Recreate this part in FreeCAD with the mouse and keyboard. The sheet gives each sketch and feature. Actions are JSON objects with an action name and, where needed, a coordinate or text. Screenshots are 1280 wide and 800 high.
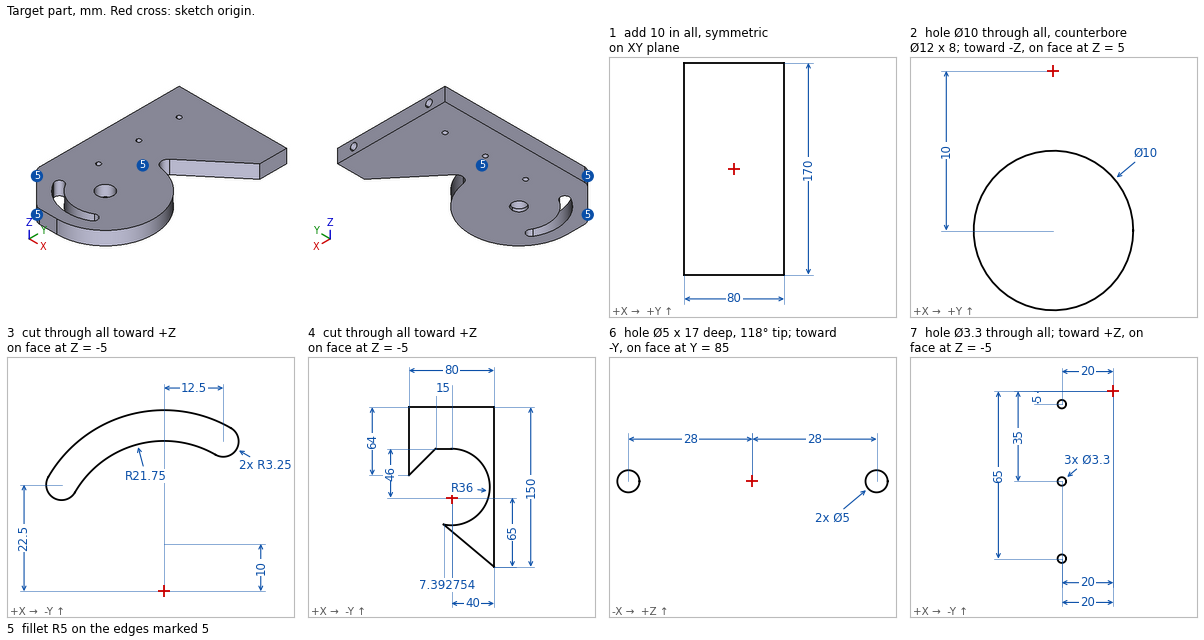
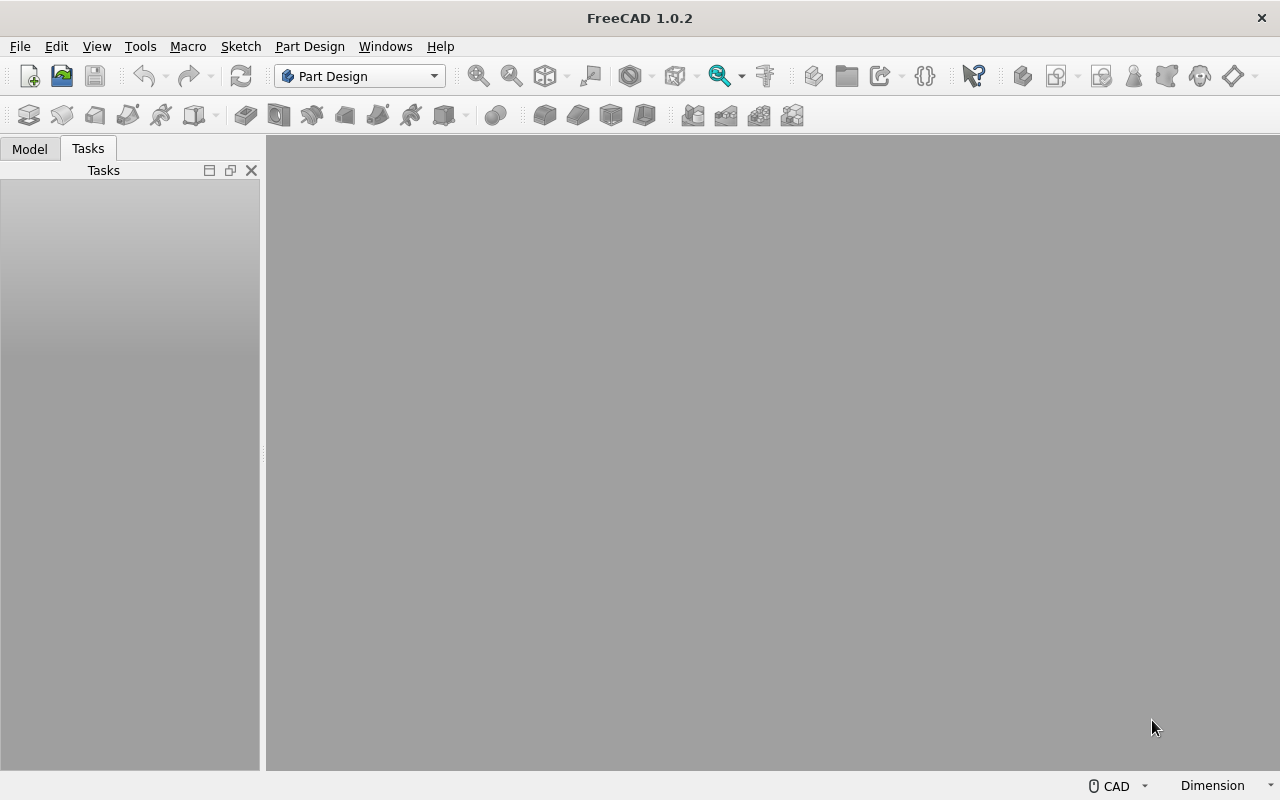
{"action": "key", "text": "ctrl+n"}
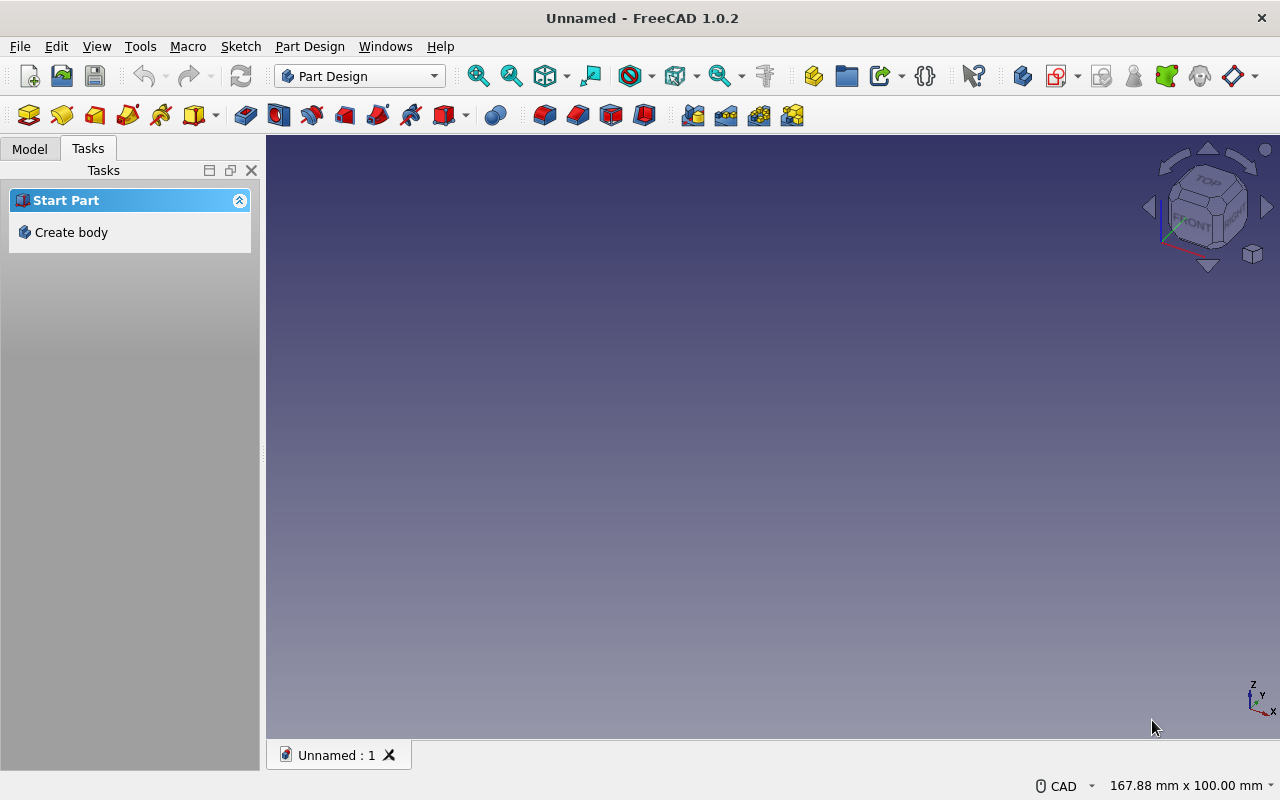
{"action": "left_click", "coordinate": [1056, 76]}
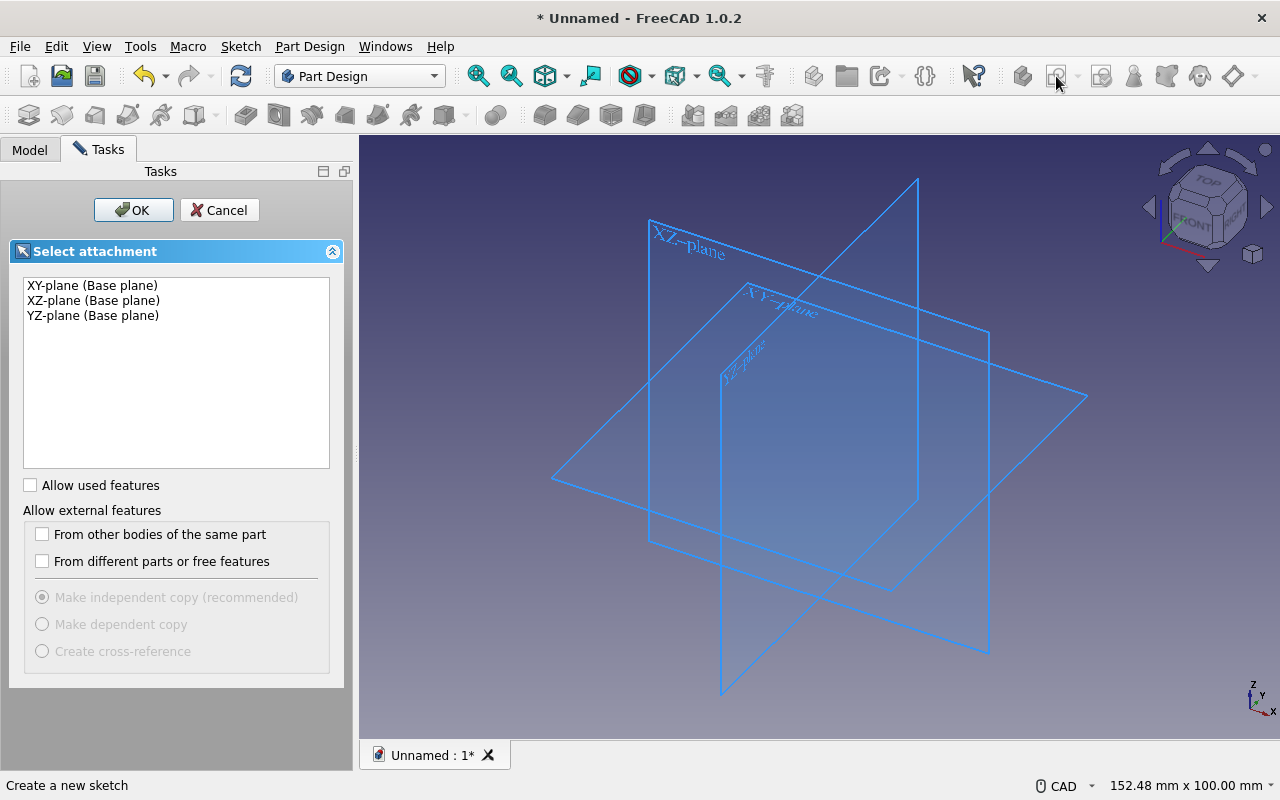
{"action": "left_click", "coordinate": [84, 286]}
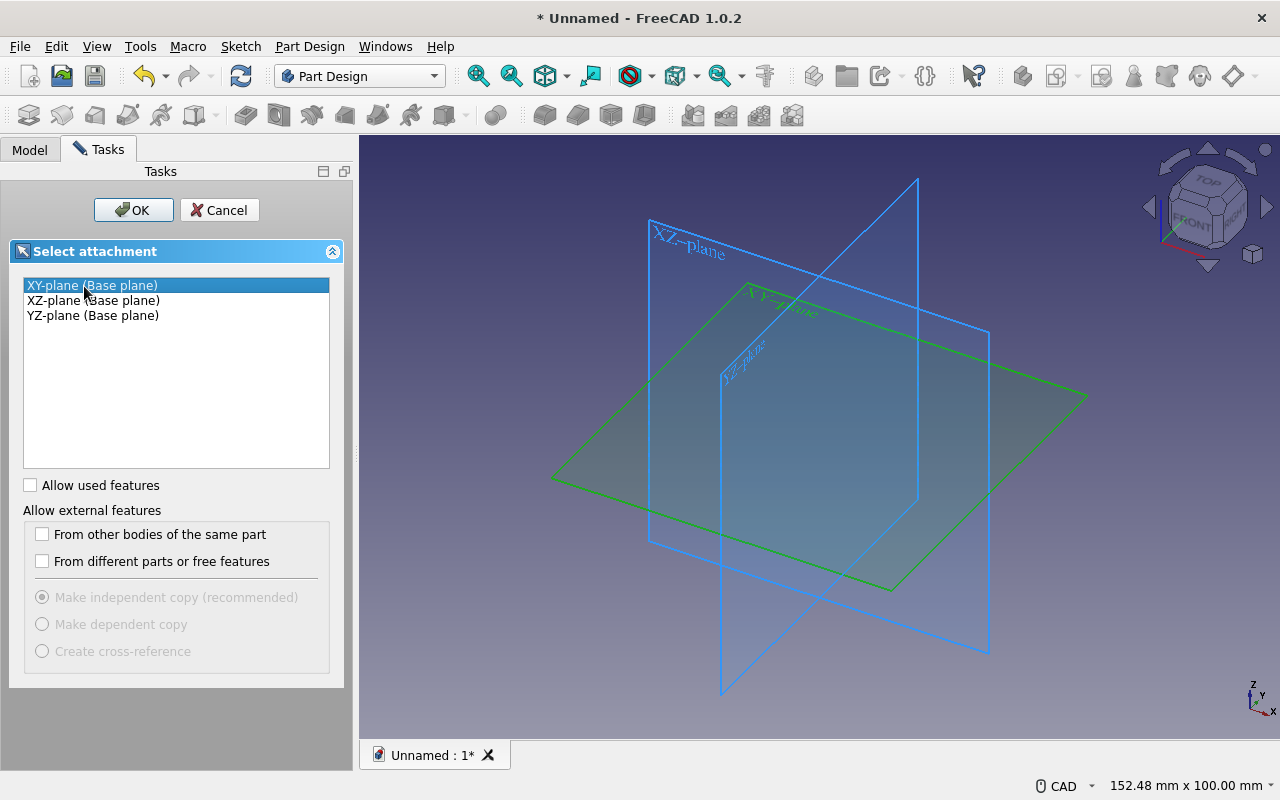
{"action": "left_click", "coordinate": [134, 210]}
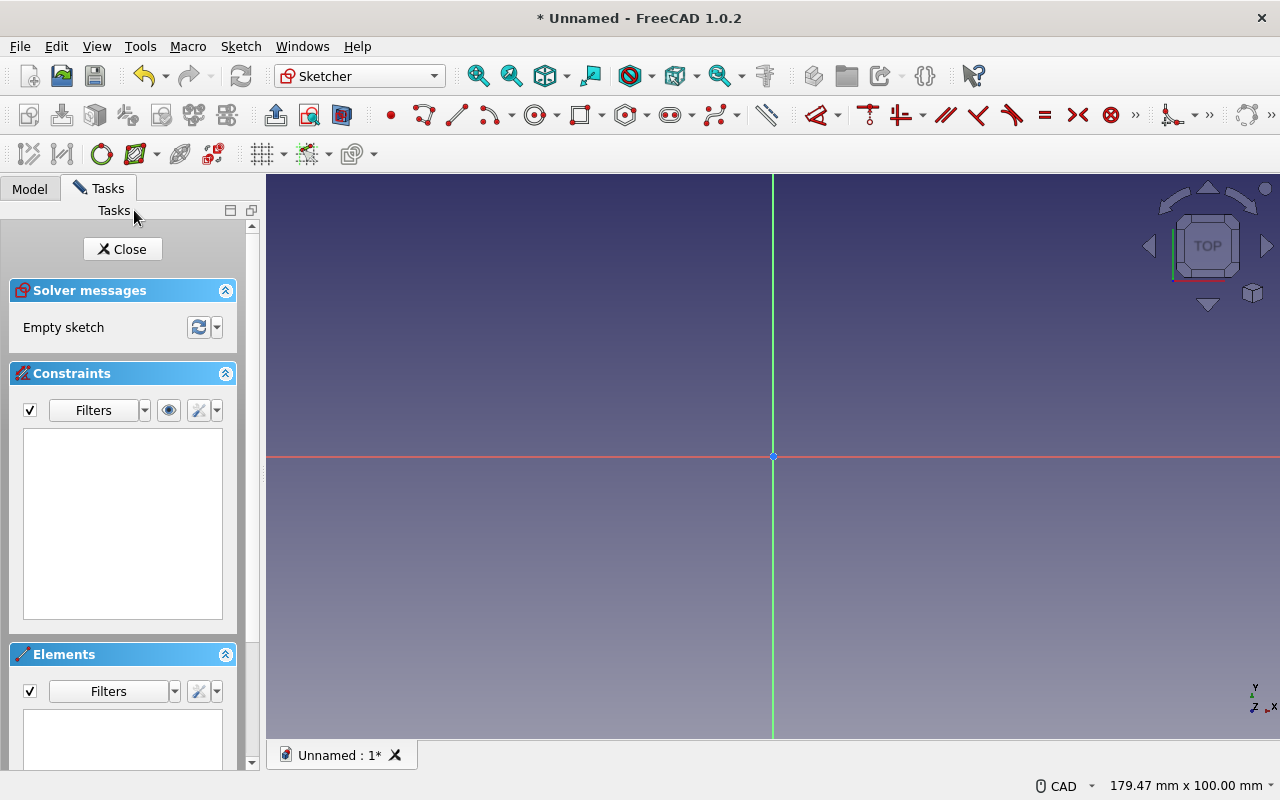
{"action": "scroll", "coordinate": [665, 456], "scroll_direction": "down", "scroll_amount": 5}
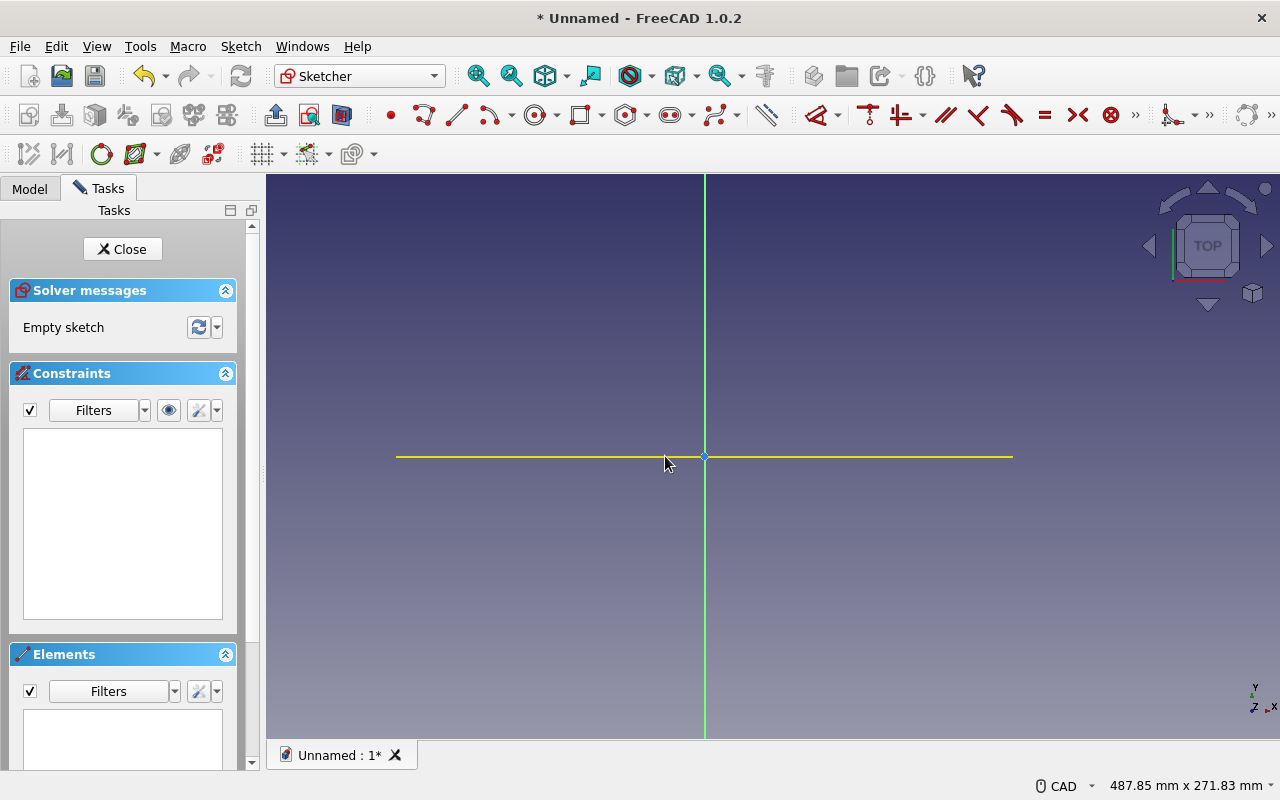
{"action": "key", "text": "g v"}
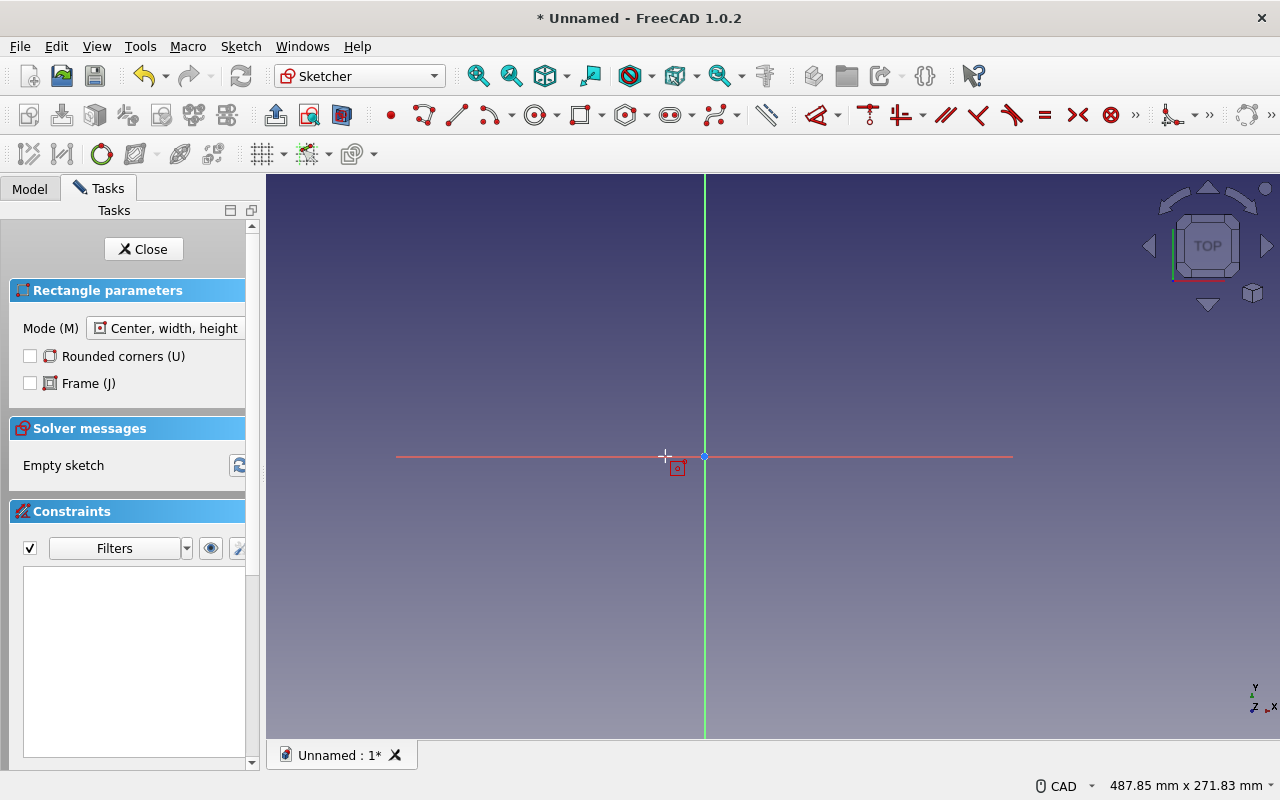
{"action": "left_click", "coordinate": [705, 456]}
{"action": "left_click", "coordinate": [788, 280]}
{"action": "key", "text": "Escape"}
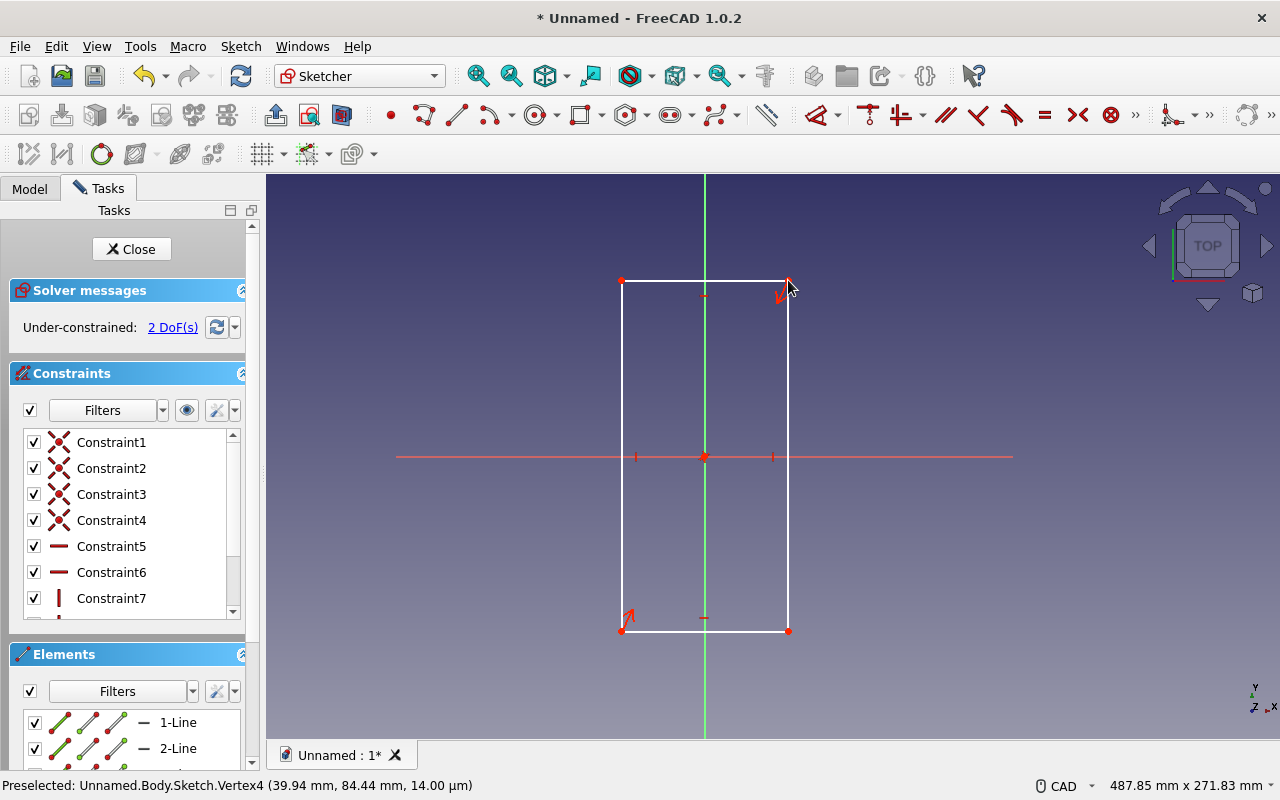
{"action": "key", "text": "d"}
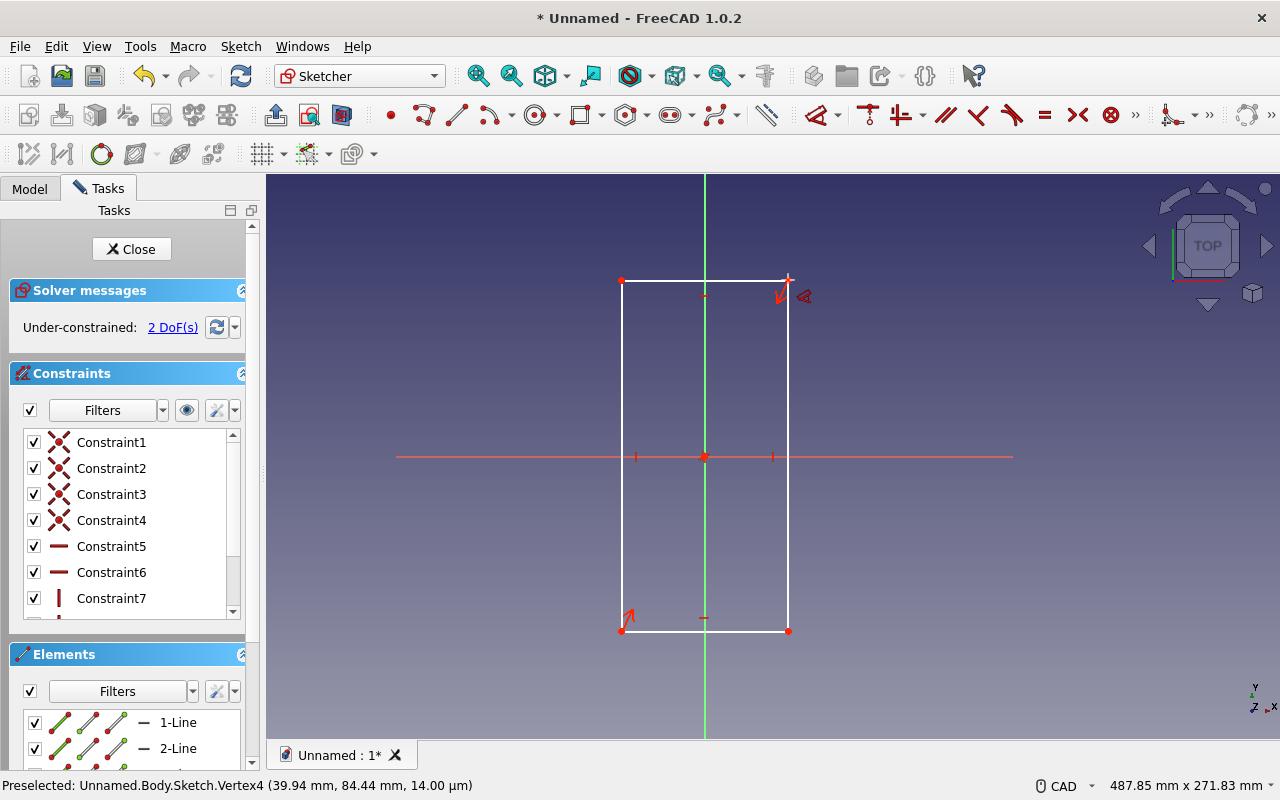
{"action": "left_click", "coordinate": [672, 632]}
{"action": "left_click", "coordinate": [667, 666]}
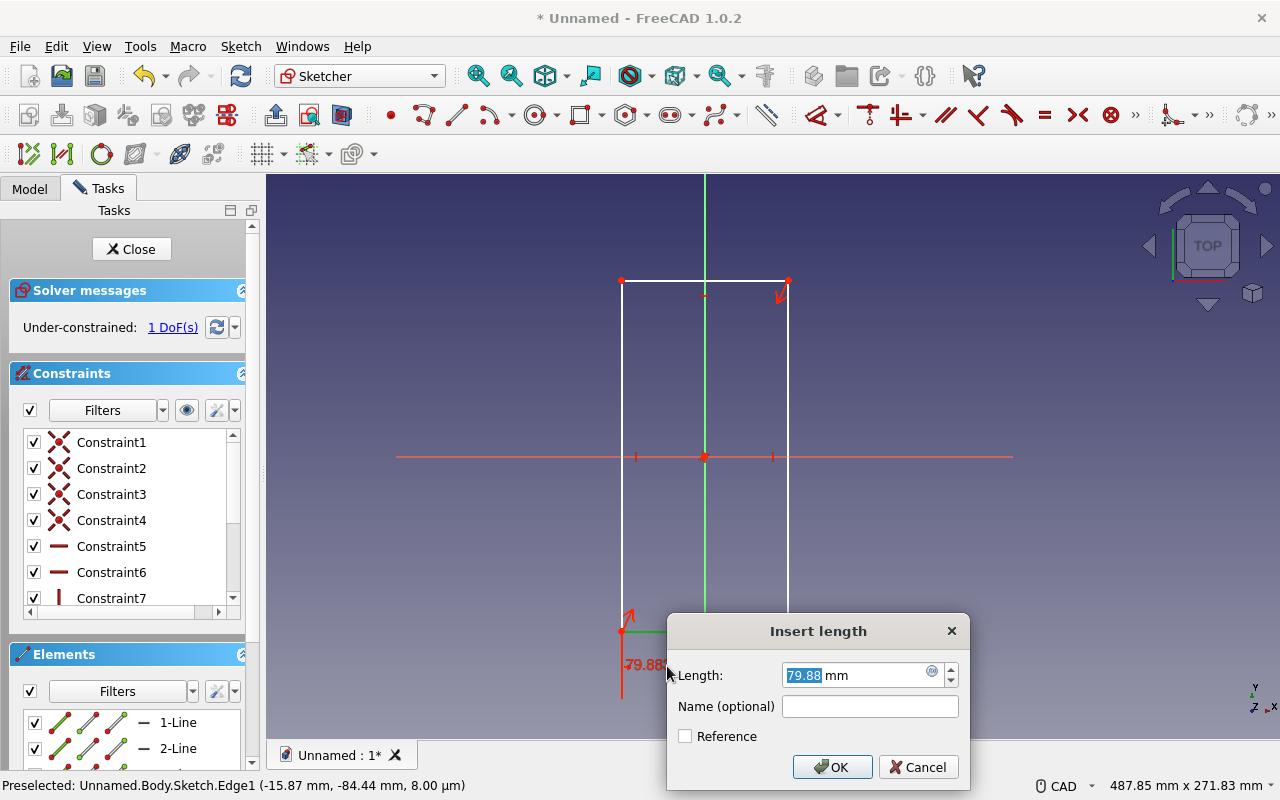
{"action": "type", "text": "80"}
{"action": "key", "text": "Return"}